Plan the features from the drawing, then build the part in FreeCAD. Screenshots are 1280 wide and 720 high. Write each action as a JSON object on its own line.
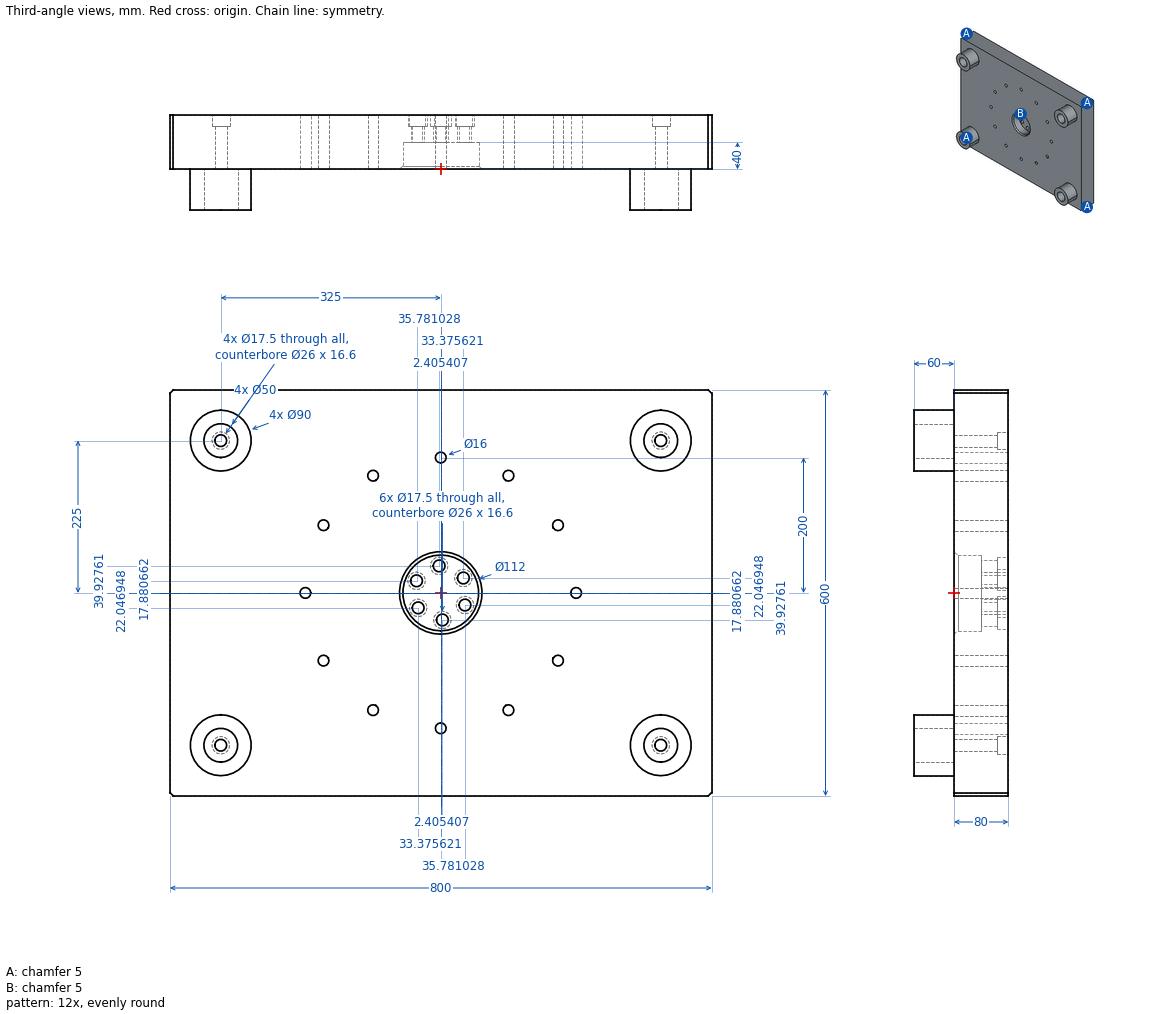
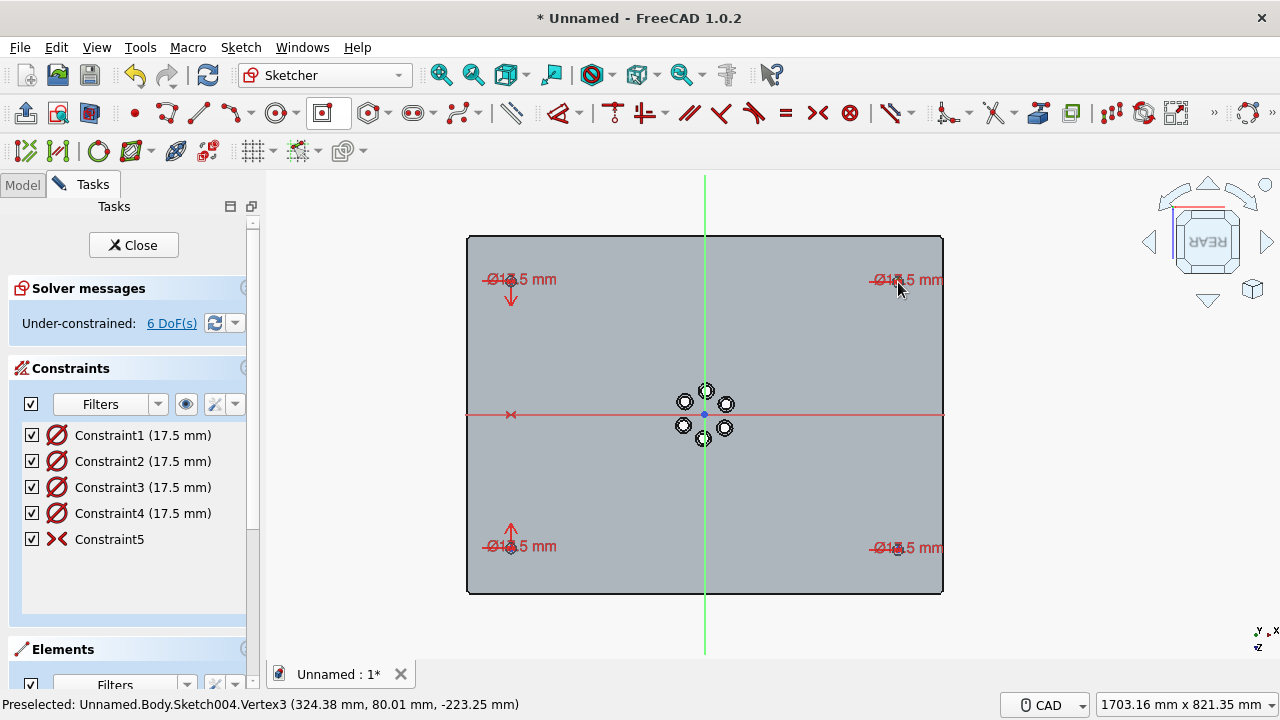
{"action": "left_click", "coordinate": [705, 600]}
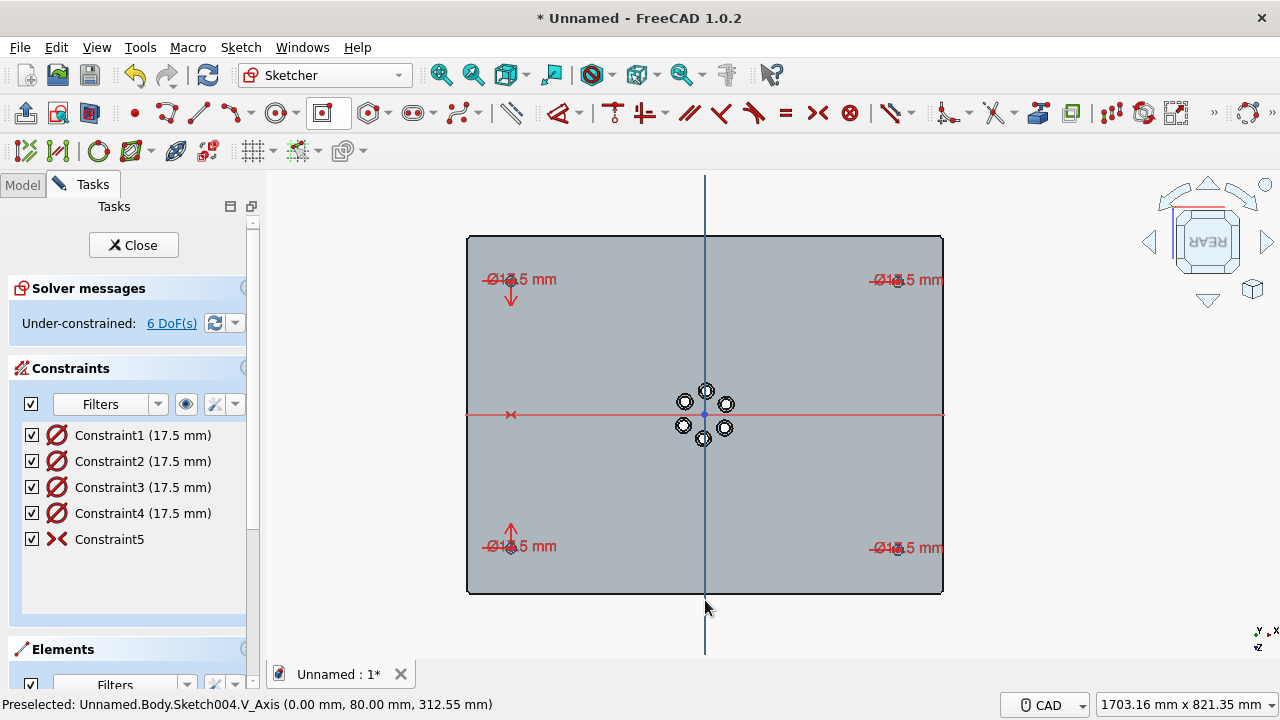
{"action": "key", "text": "s"}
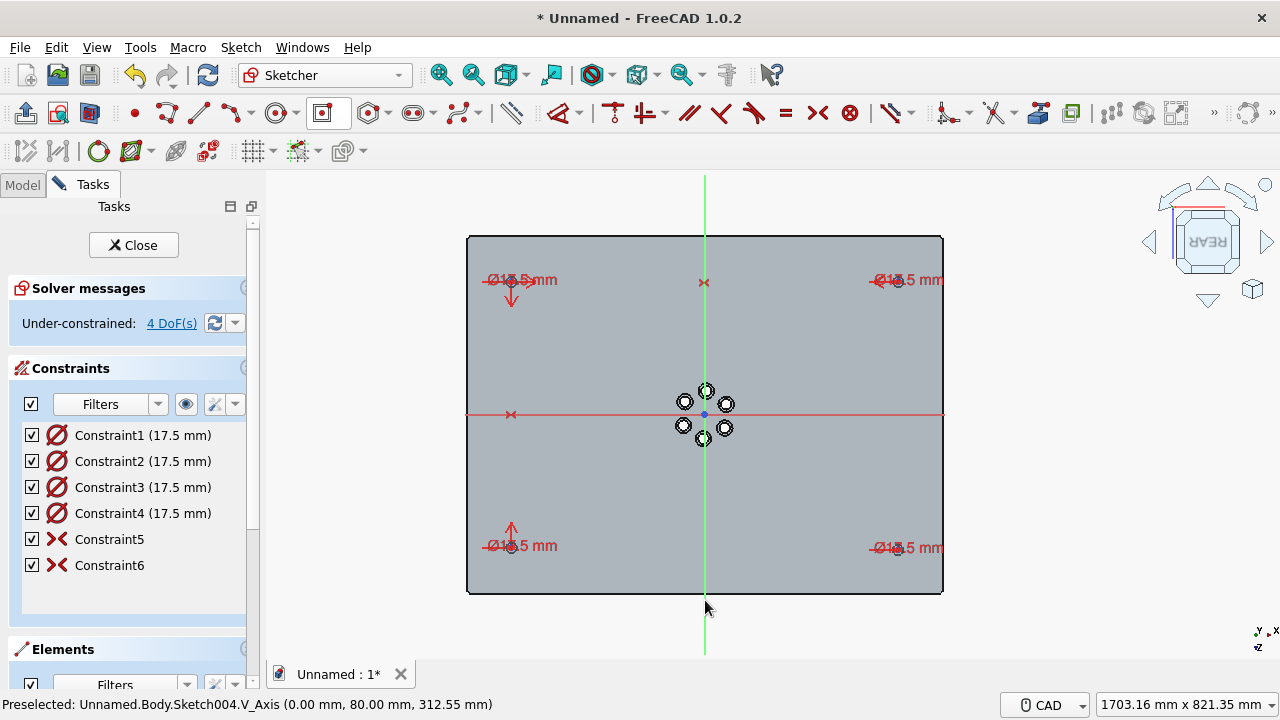
{"action": "left_click", "coordinate": [511, 548]}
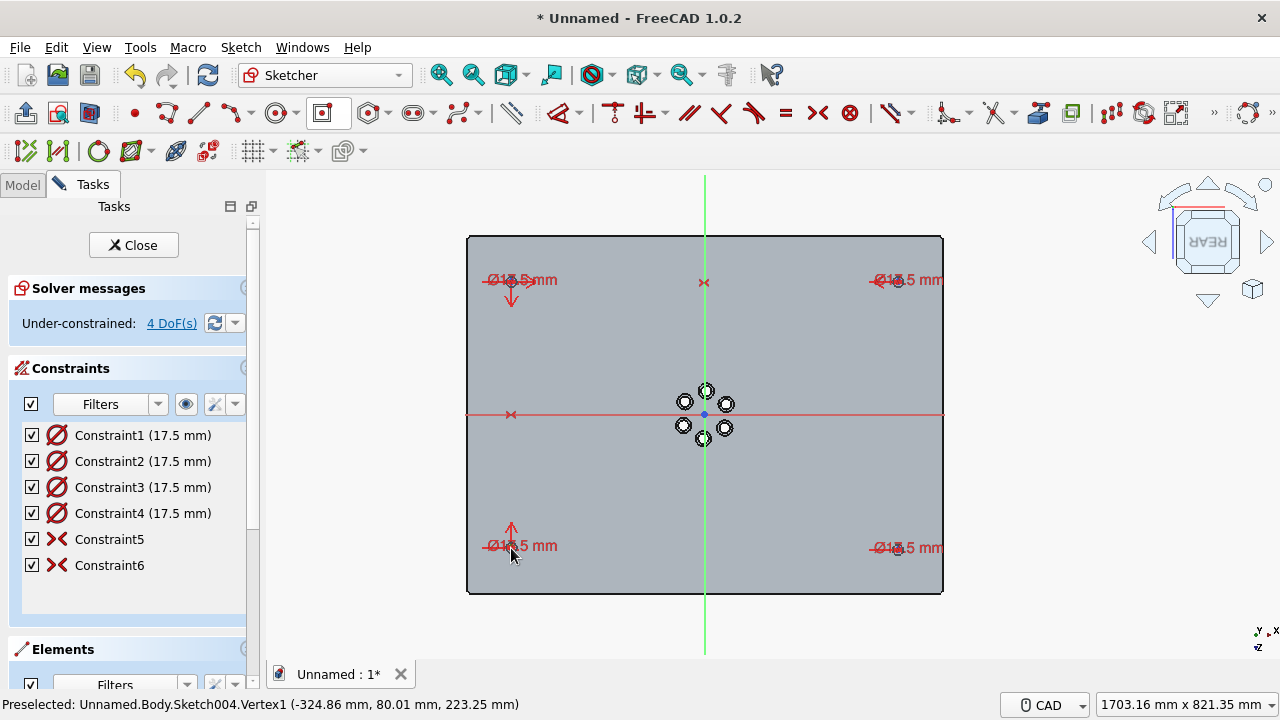
{"action": "left_click", "coordinate": [898, 550]}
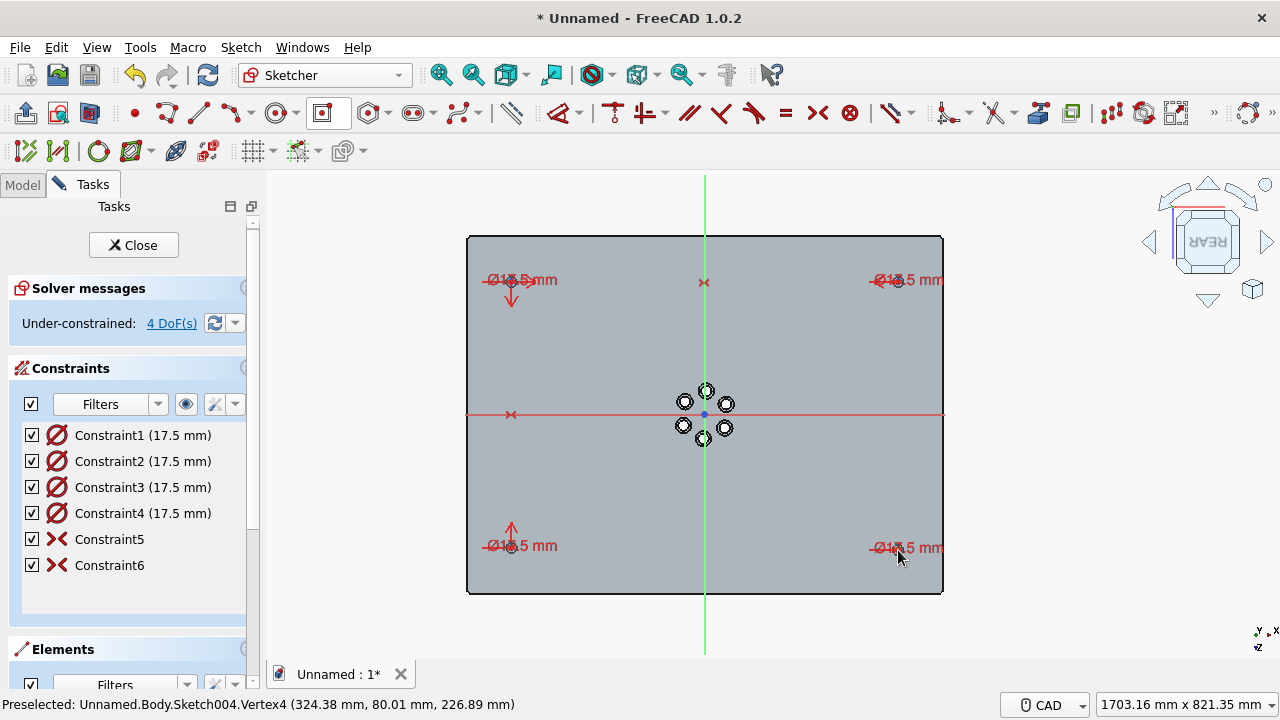
{"action": "left_click", "coordinate": [705, 600]}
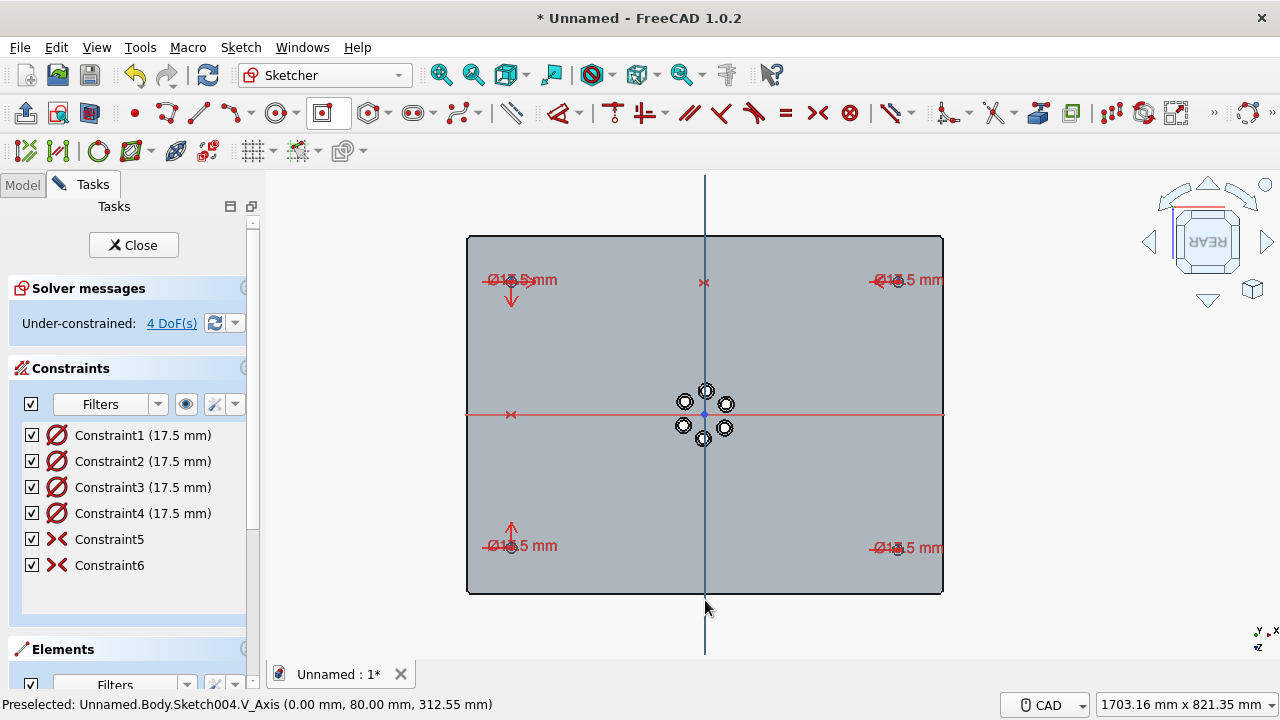
{"action": "key", "text": "s"}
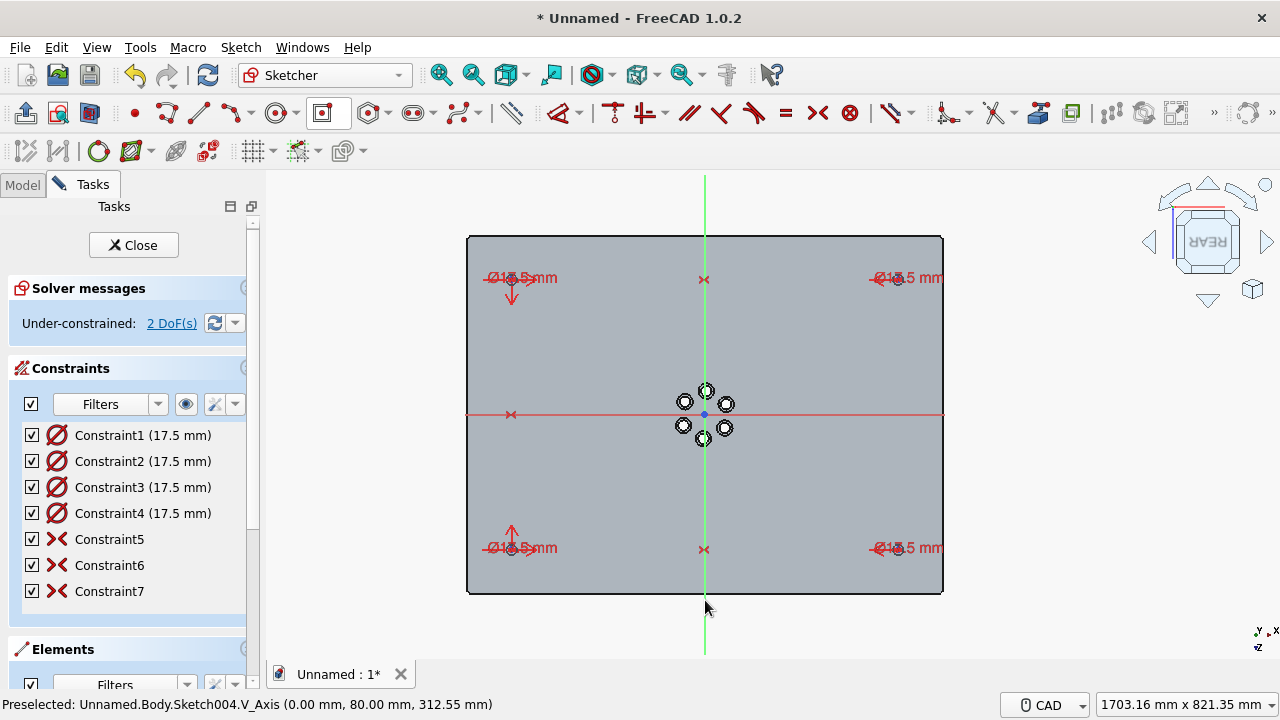
{"action": "left_click", "coordinate": [512, 550]}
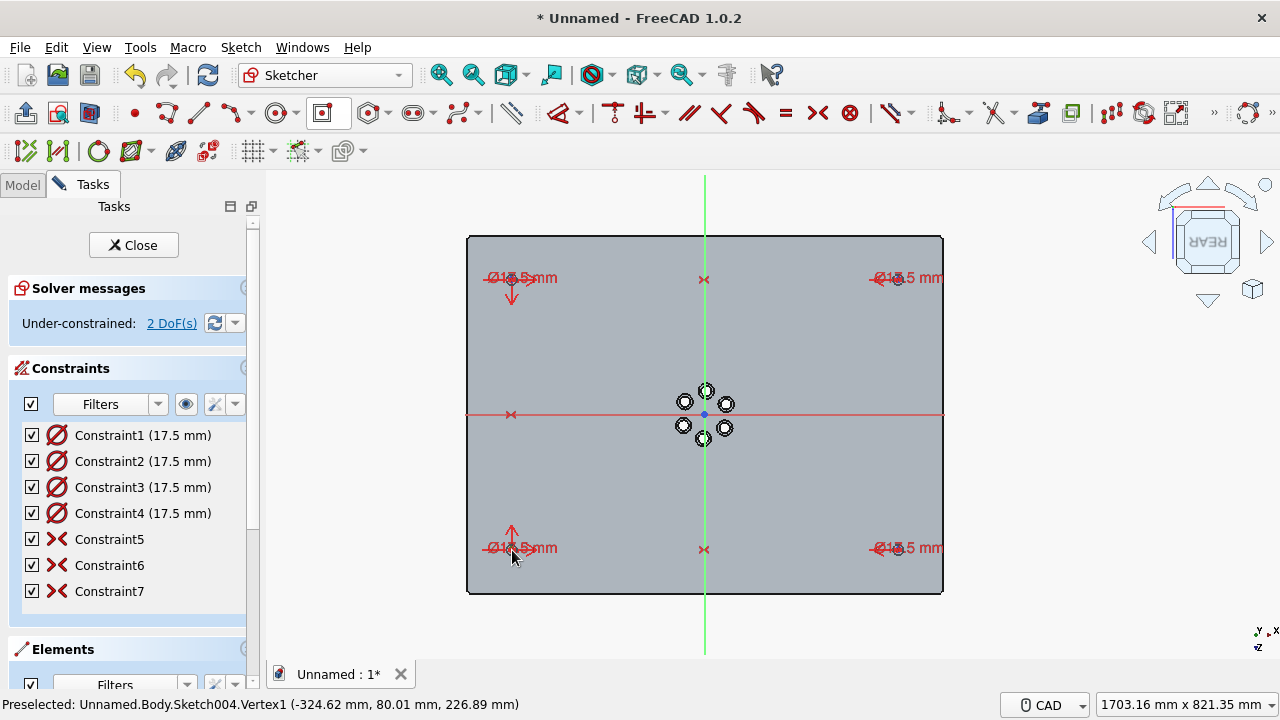
{"action": "left_click", "coordinate": [582, 114]}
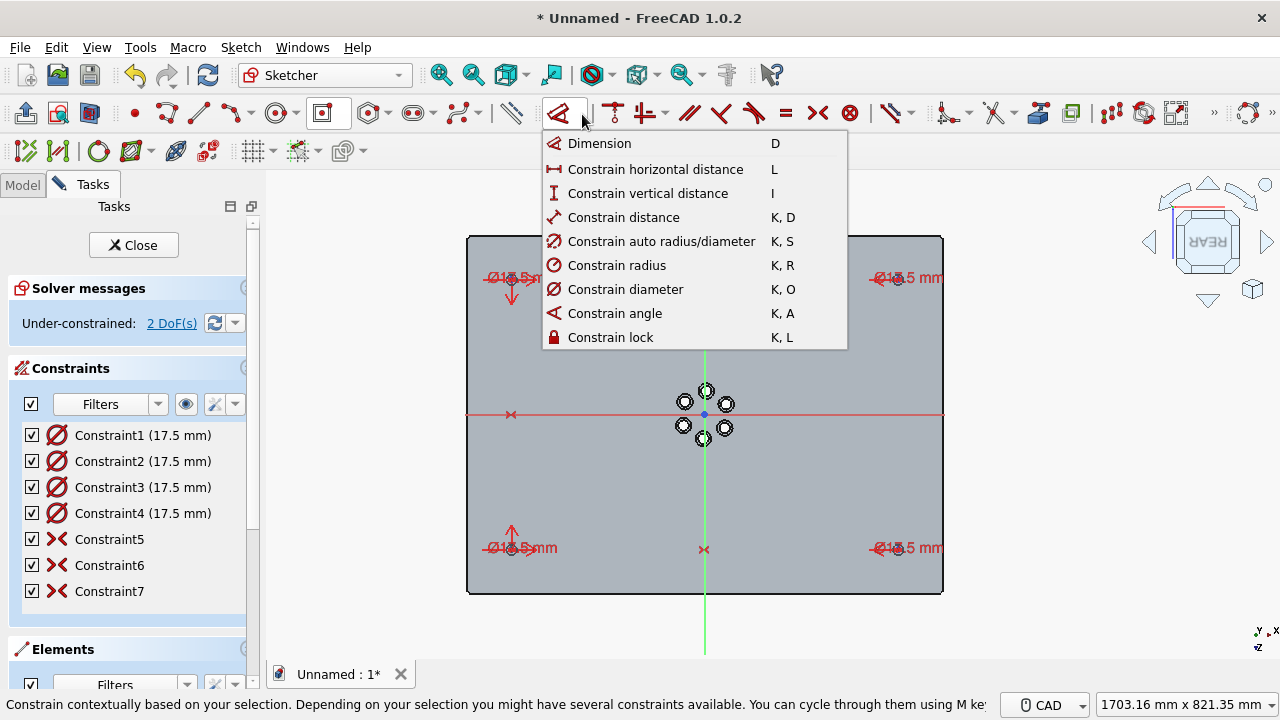
{"action": "left_click", "coordinate": [695, 169]}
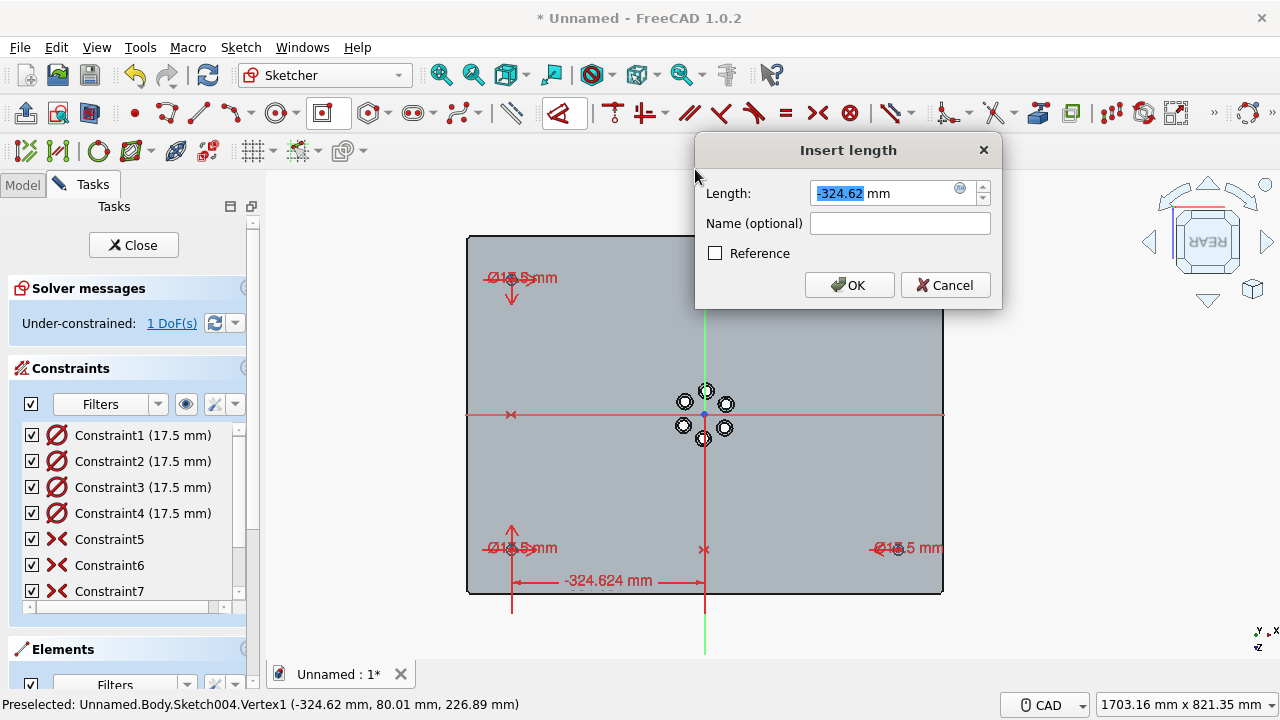
{"action": "type", "text": "-325"}
{"action": "key", "text": "Return"}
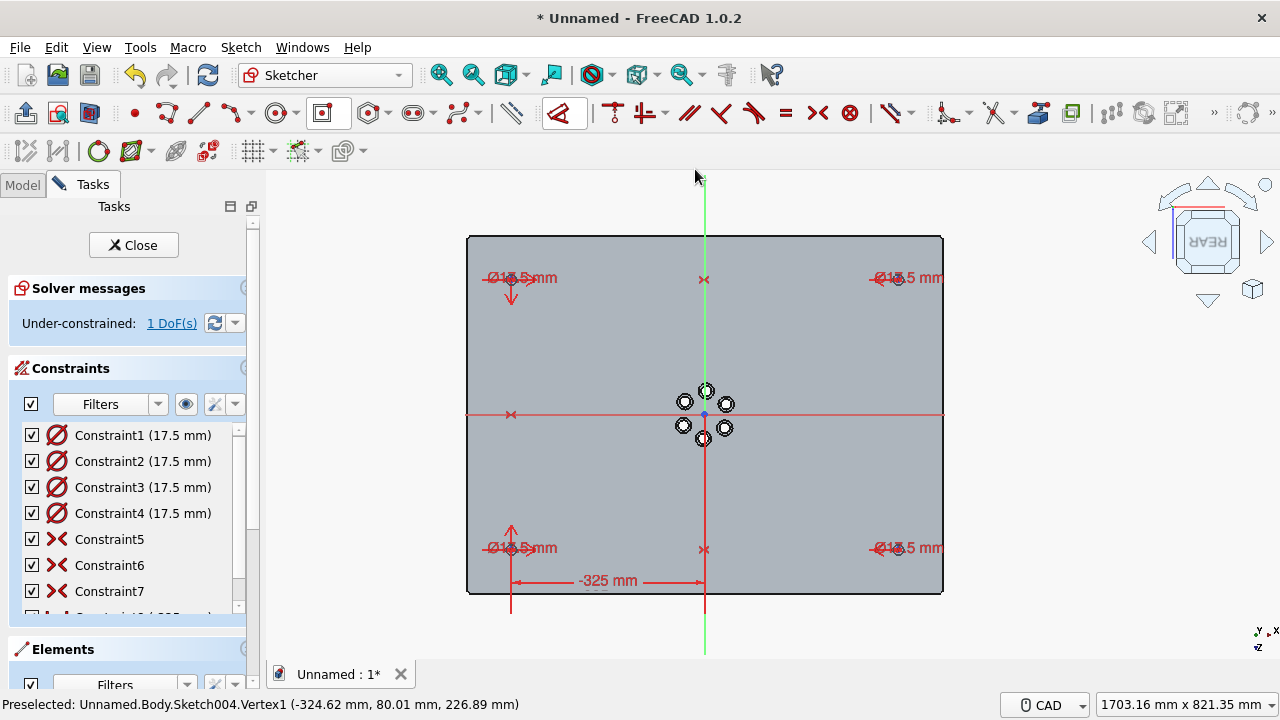
{"action": "left_click", "coordinate": [511, 550]}